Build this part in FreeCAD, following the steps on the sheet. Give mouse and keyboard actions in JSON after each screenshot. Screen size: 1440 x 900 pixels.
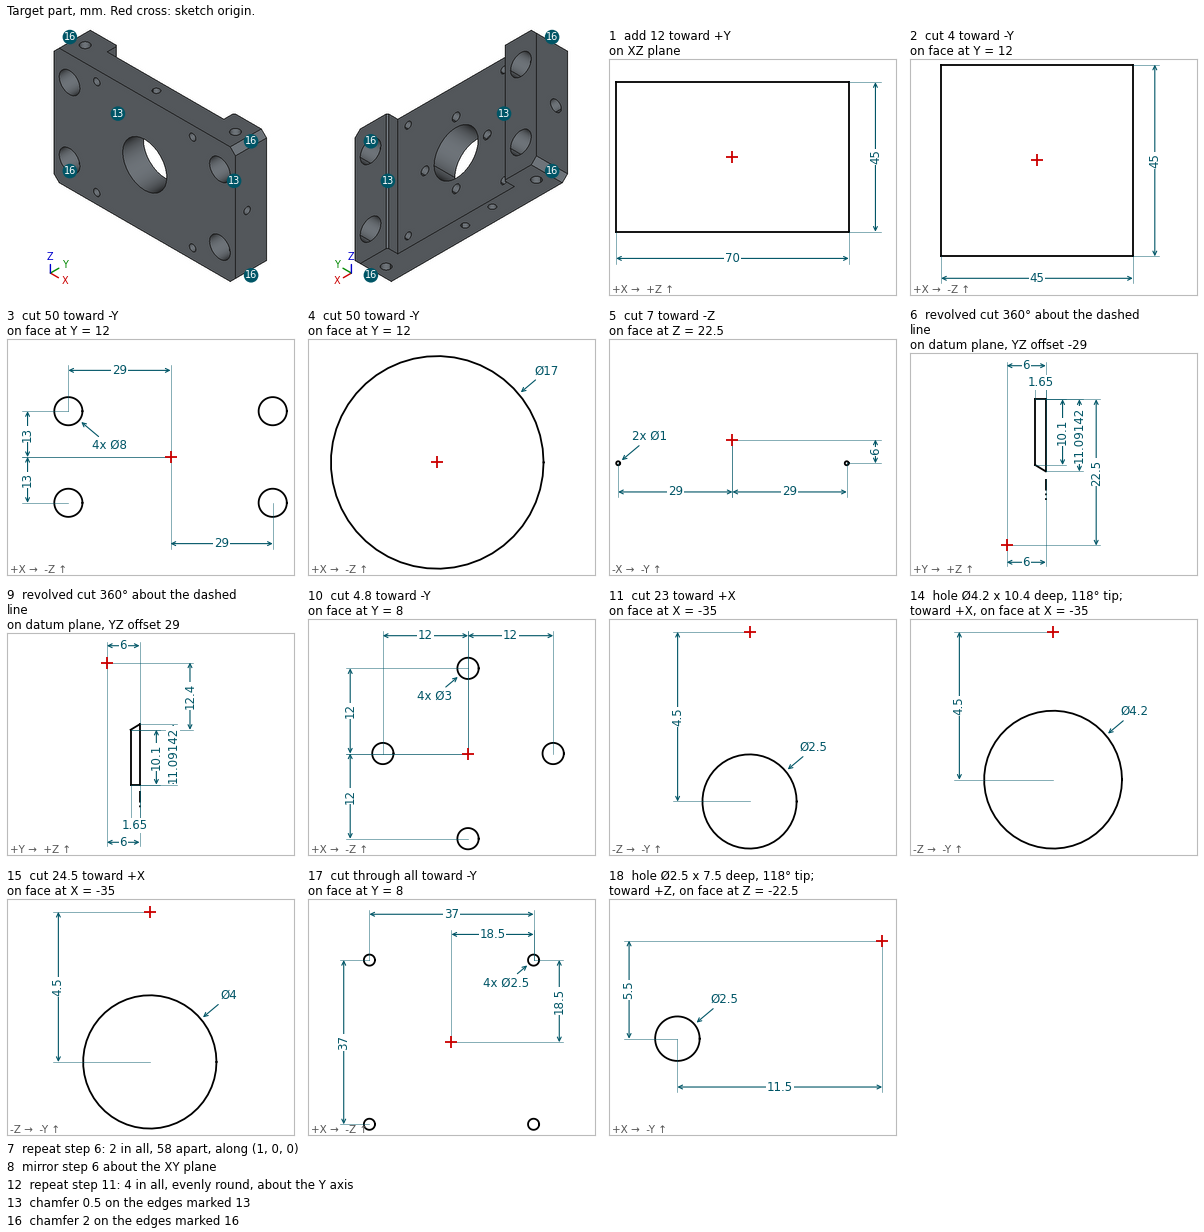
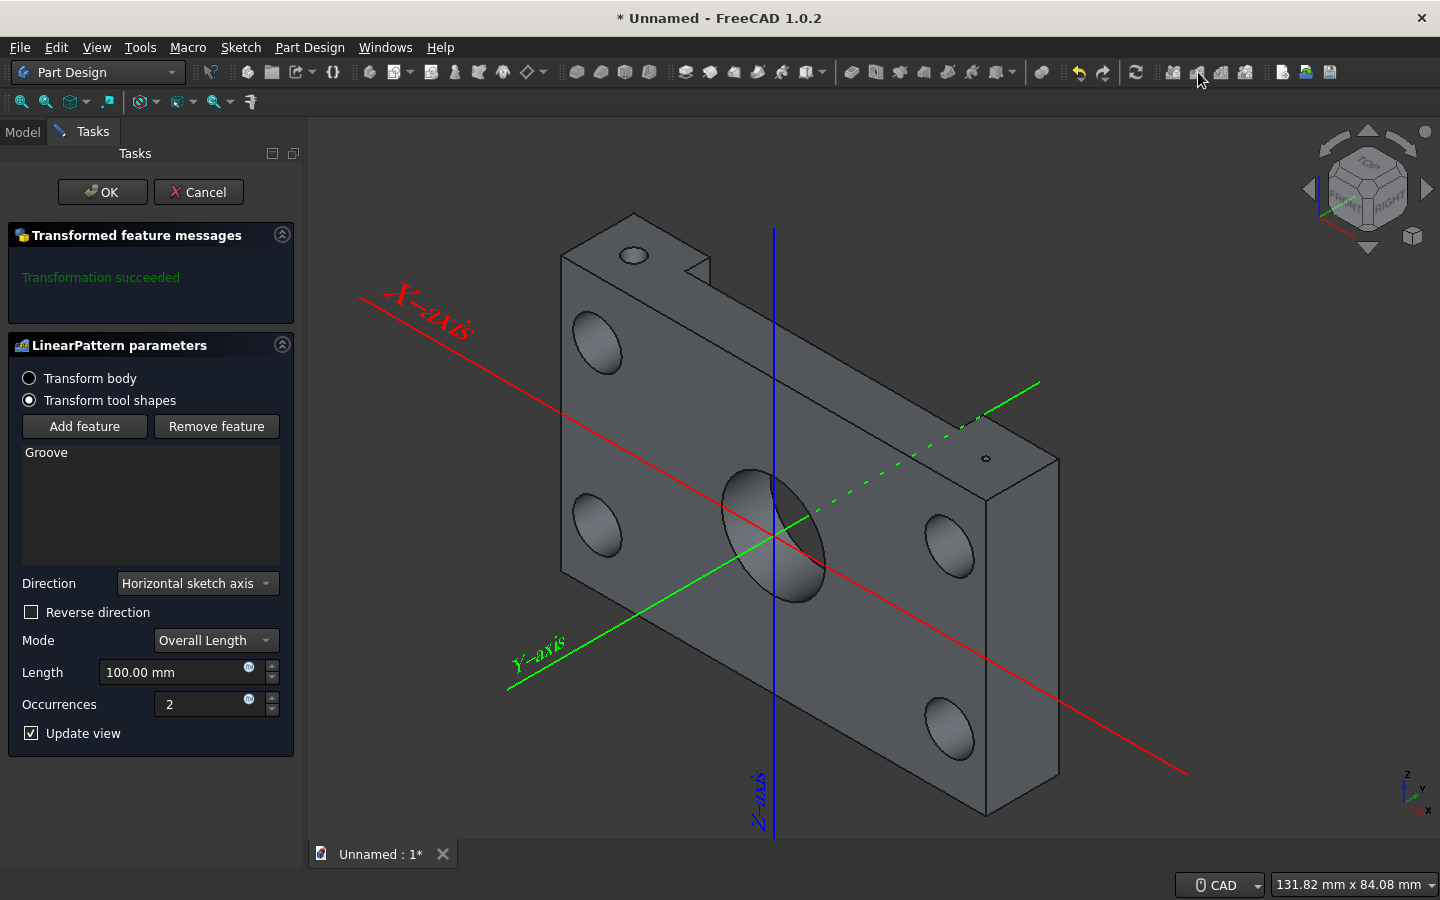
{"action": "left_click", "coordinate": [198, 584]}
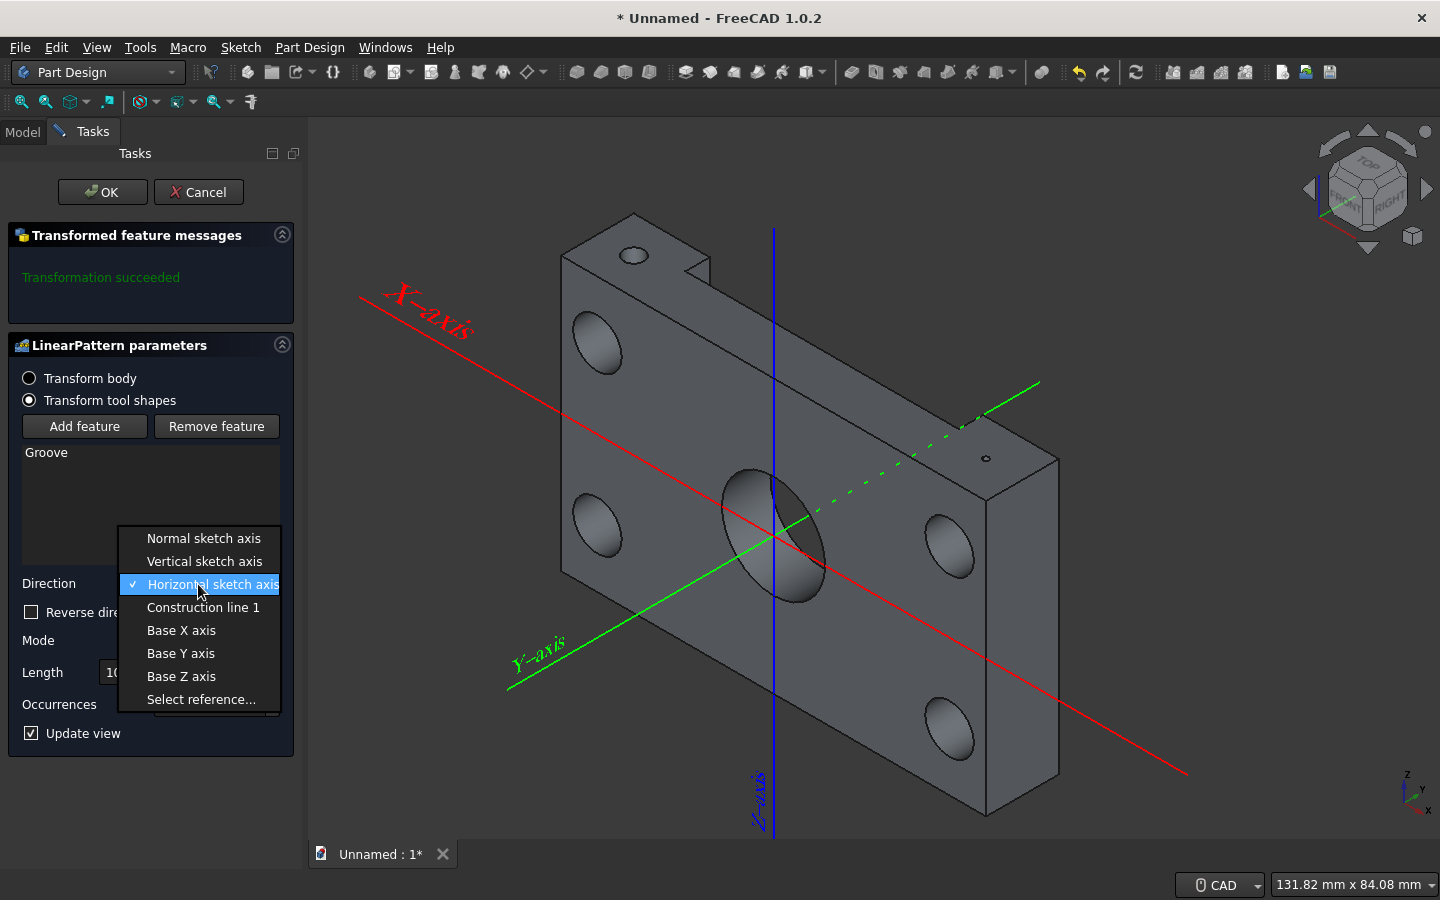
{"action": "left_click", "coordinate": [198, 630]}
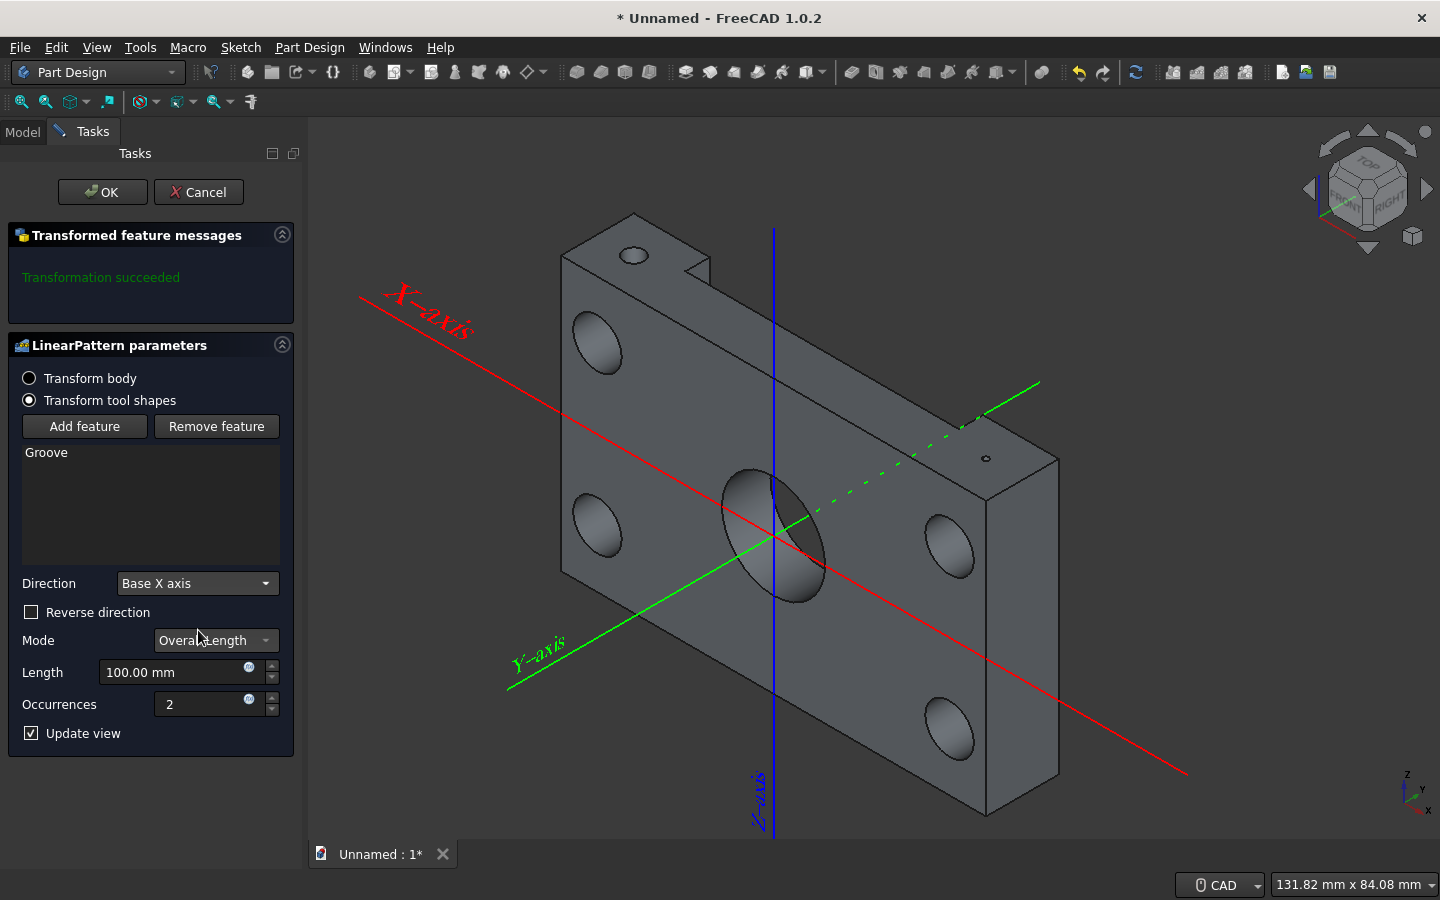
{"action": "left_click", "coordinate": [217, 640]}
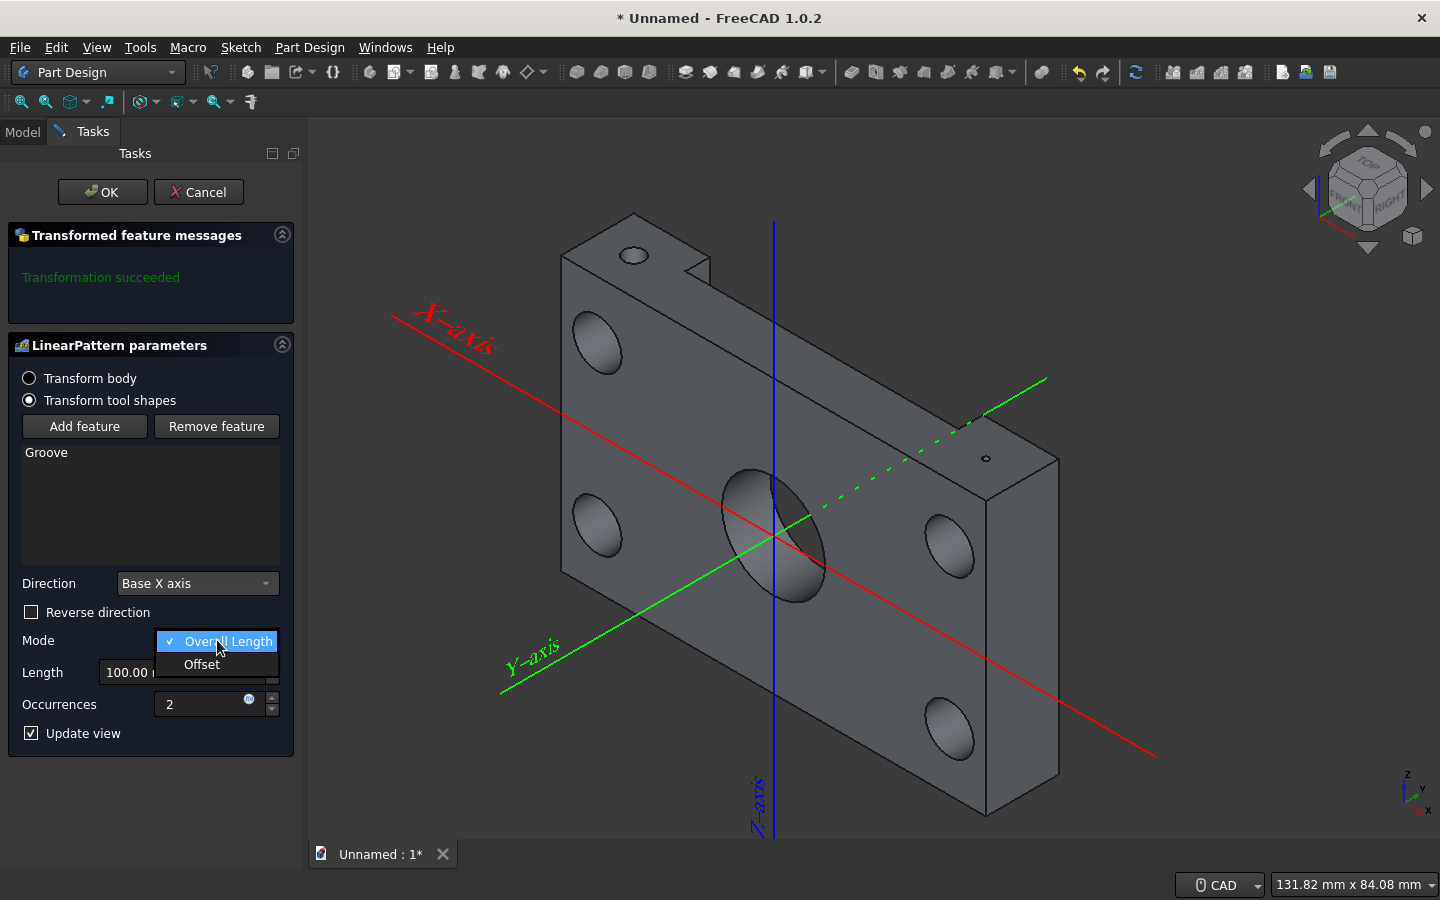
{"action": "left_click", "coordinate": [216, 664]}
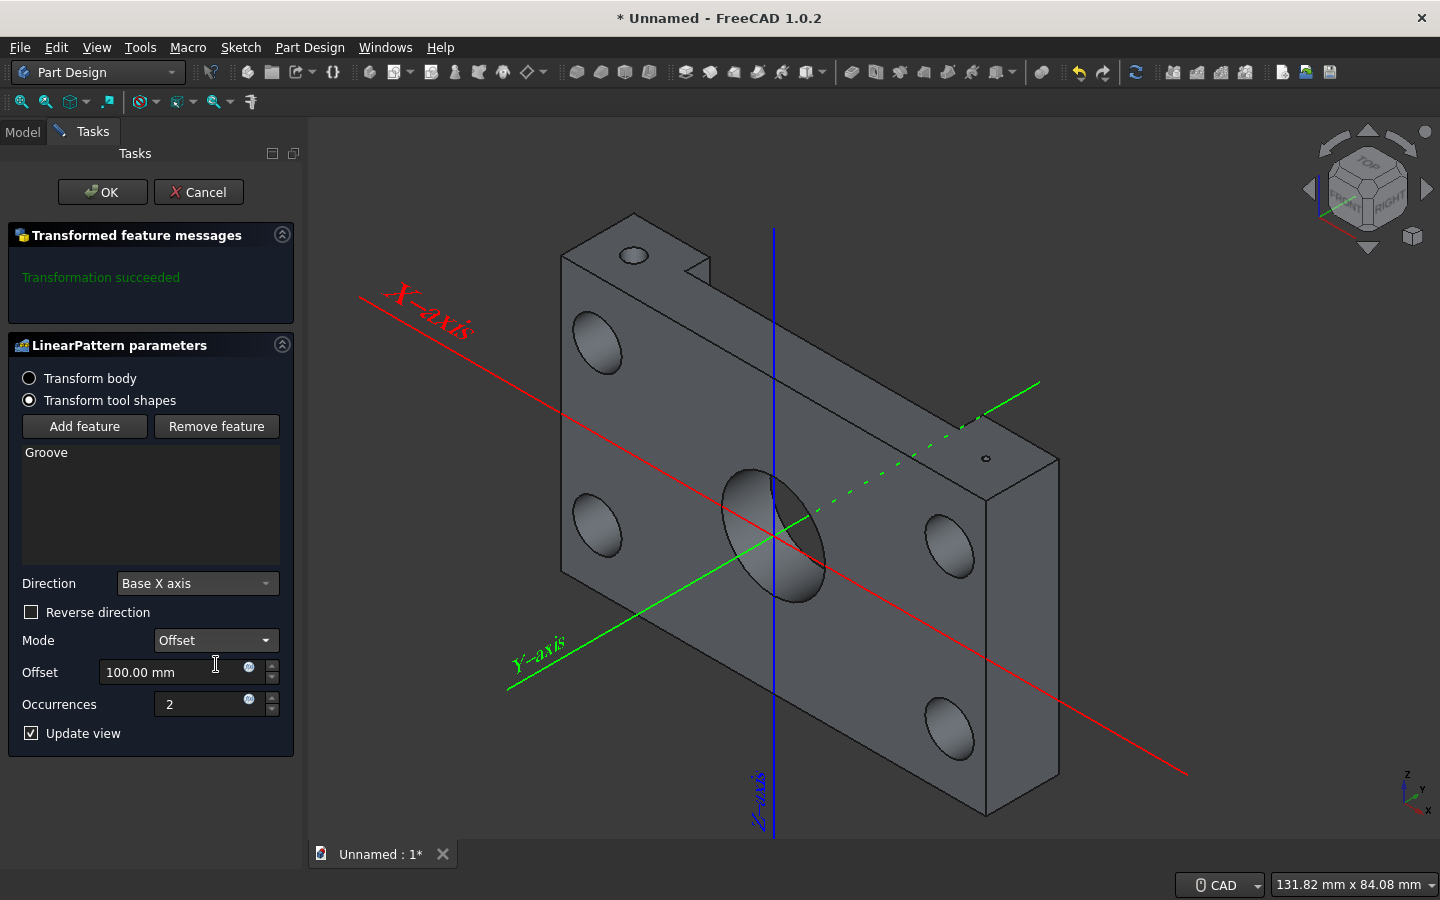
{"action": "triple_click", "coordinate": [182, 672]}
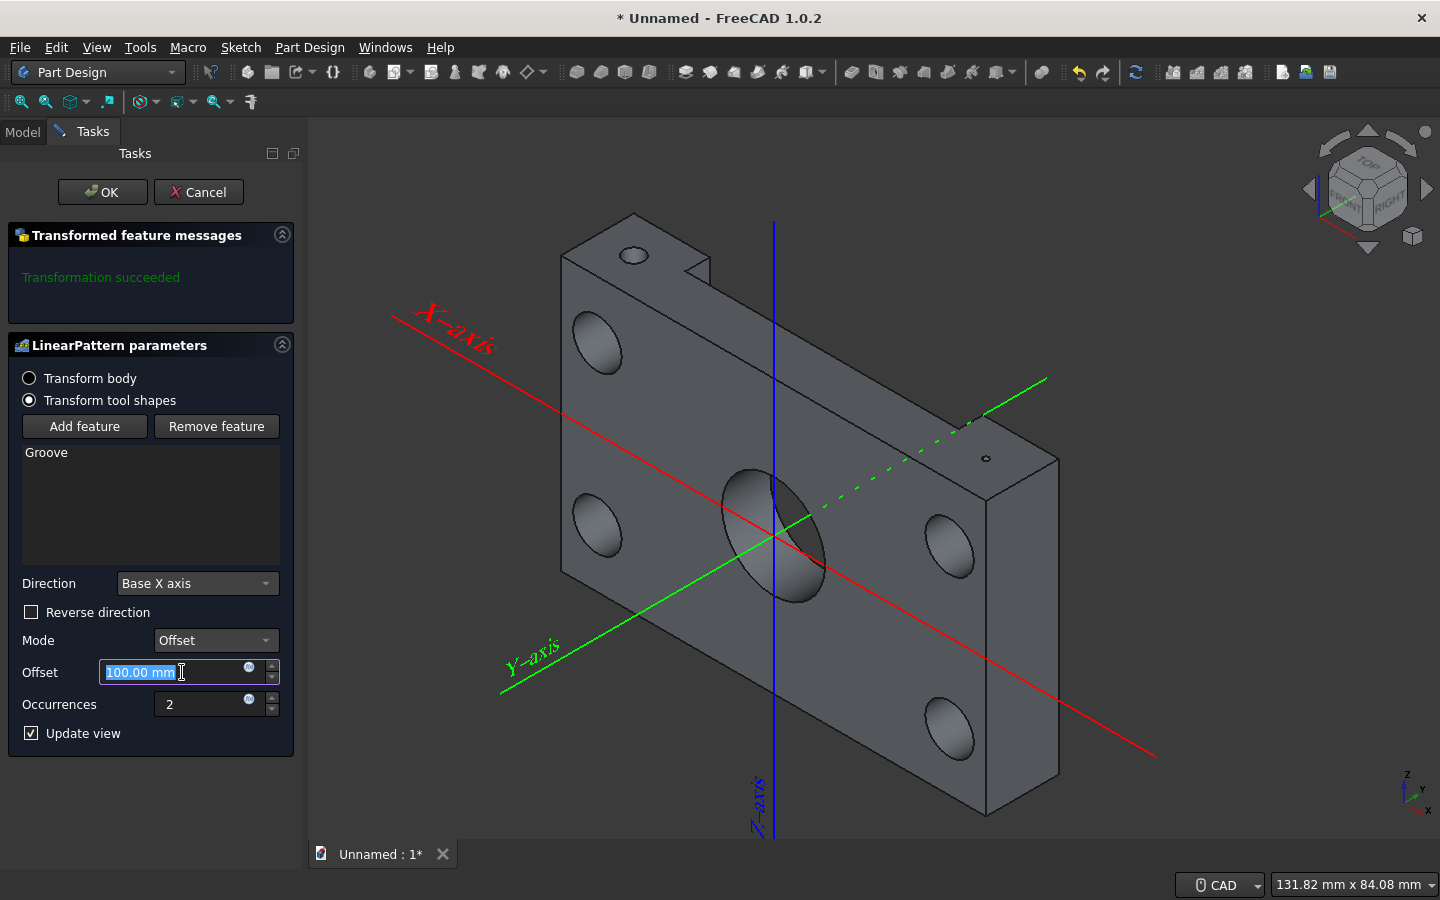
{"action": "type", "text": "58"}
{"action": "key", "text": "Tab"}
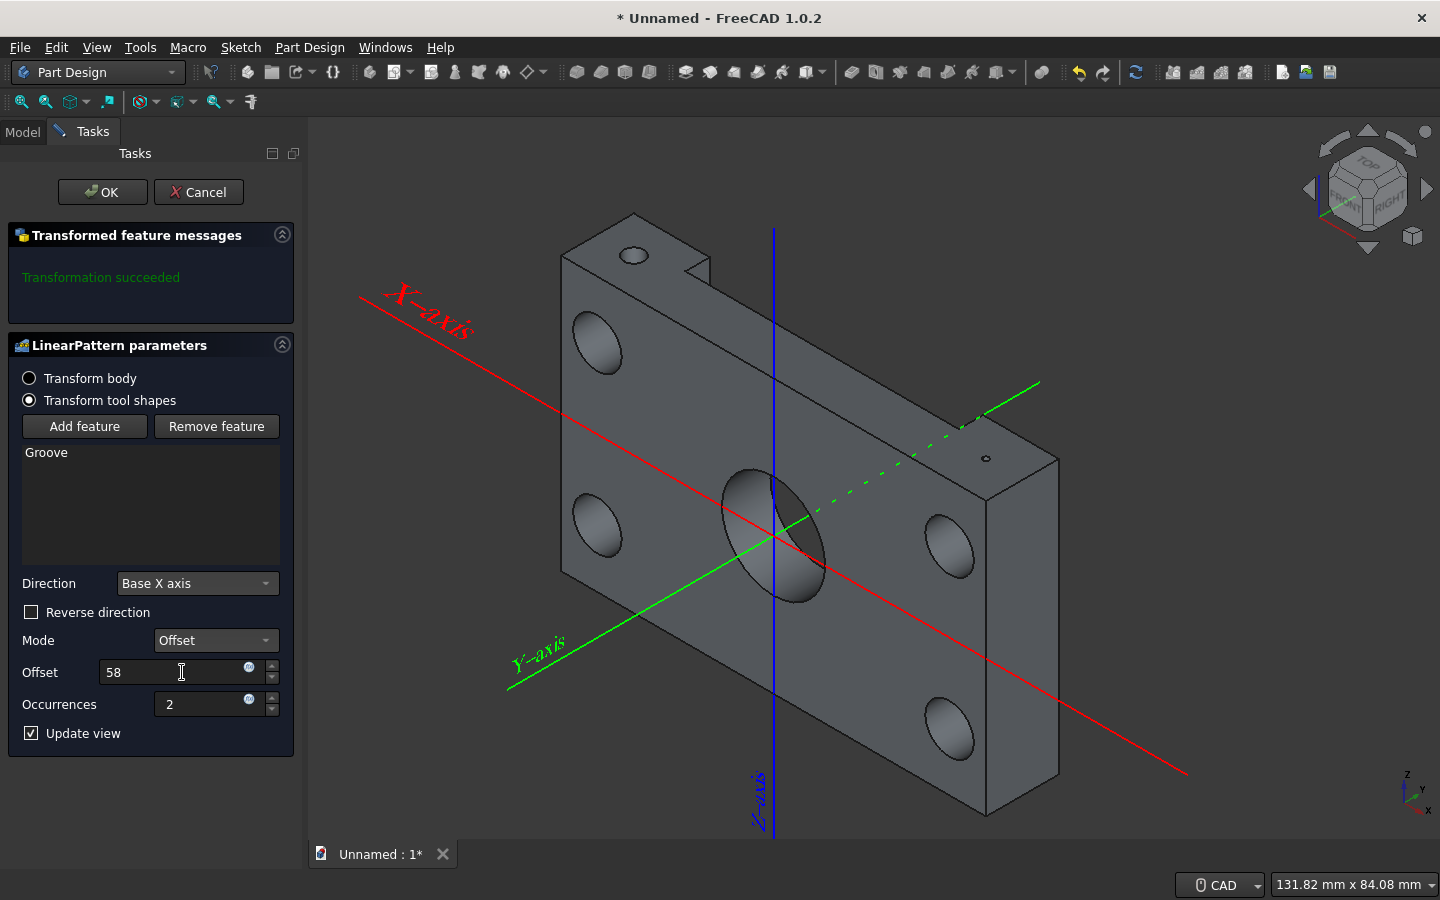
{"action": "triple_click", "coordinate": [209, 704]}